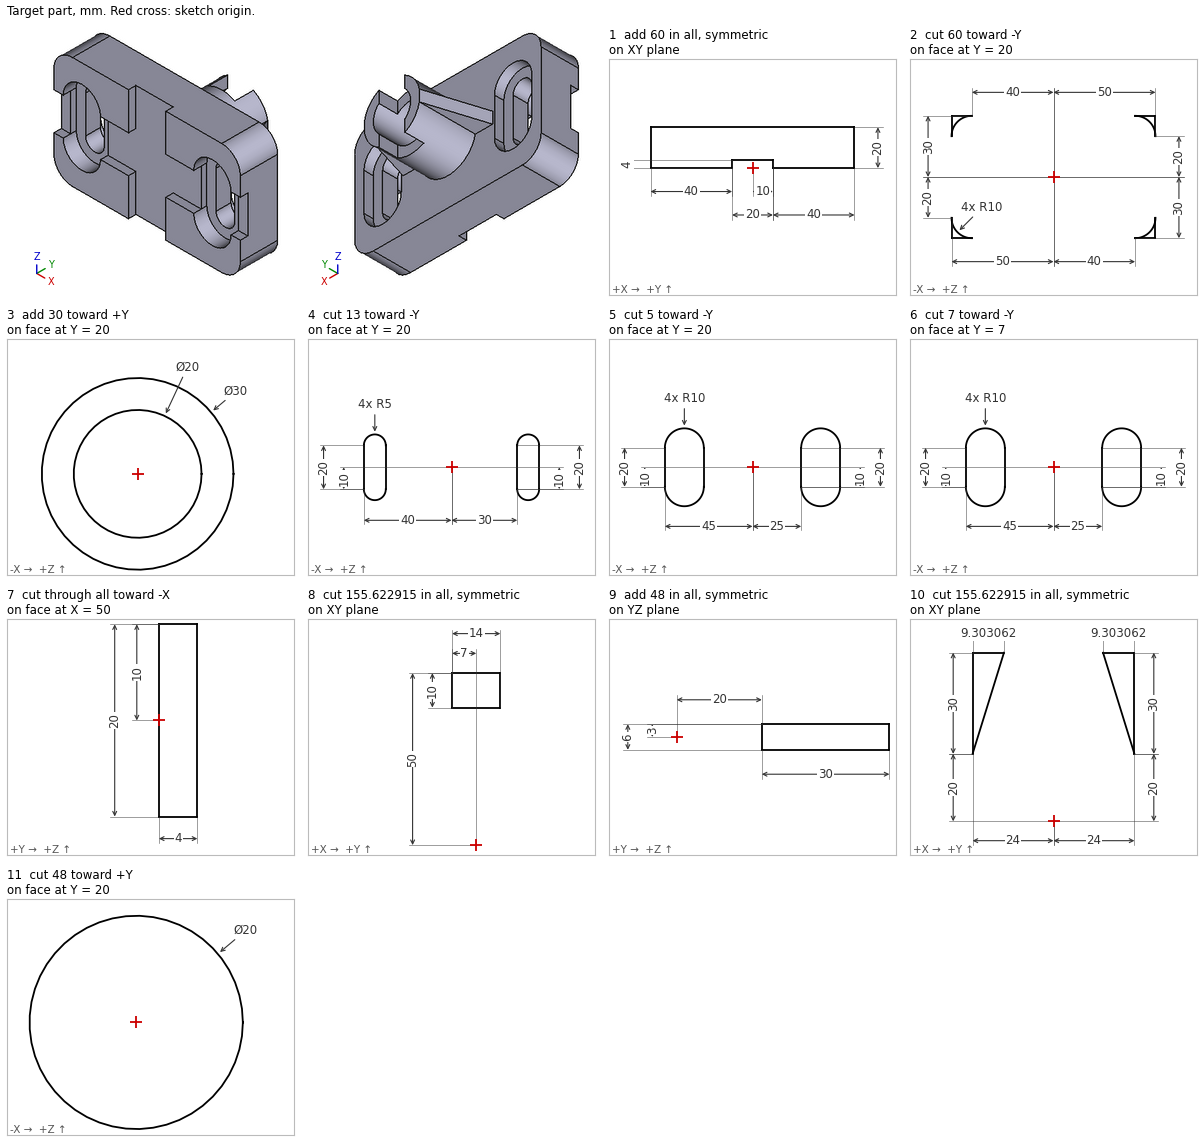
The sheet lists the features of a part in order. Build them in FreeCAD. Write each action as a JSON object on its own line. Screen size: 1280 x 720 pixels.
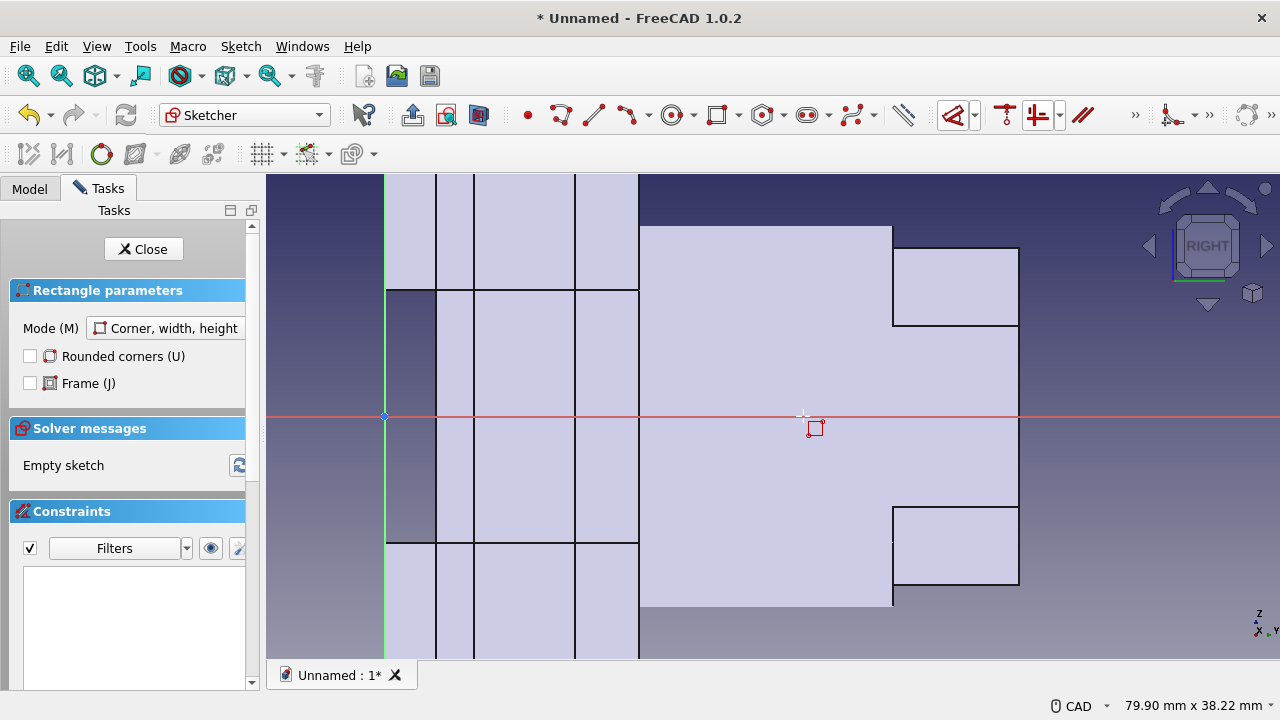
{"action": "left_click", "coordinate": [639, 378]}
{"action": "left_click", "coordinate": [1019, 455]}
{"action": "key", "text": "Escape"}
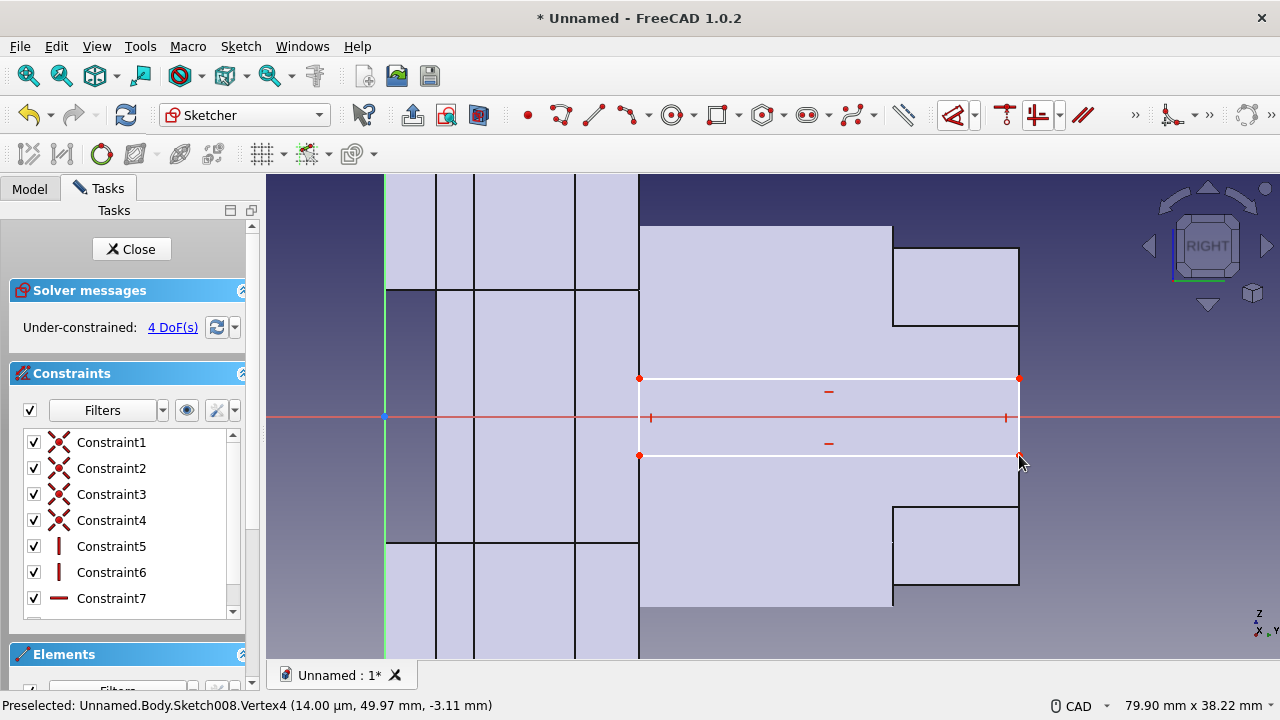
{"action": "left_click", "coordinate": [639, 402]}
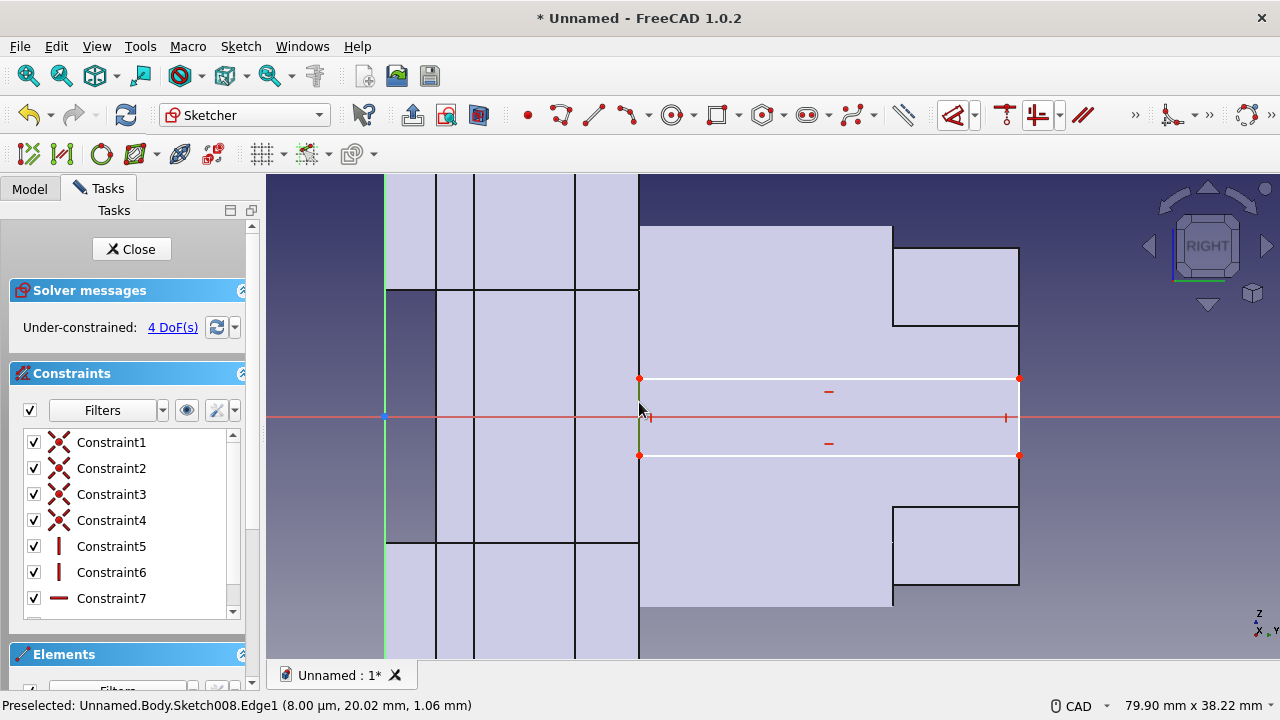
{"action": "key", "text": "i"}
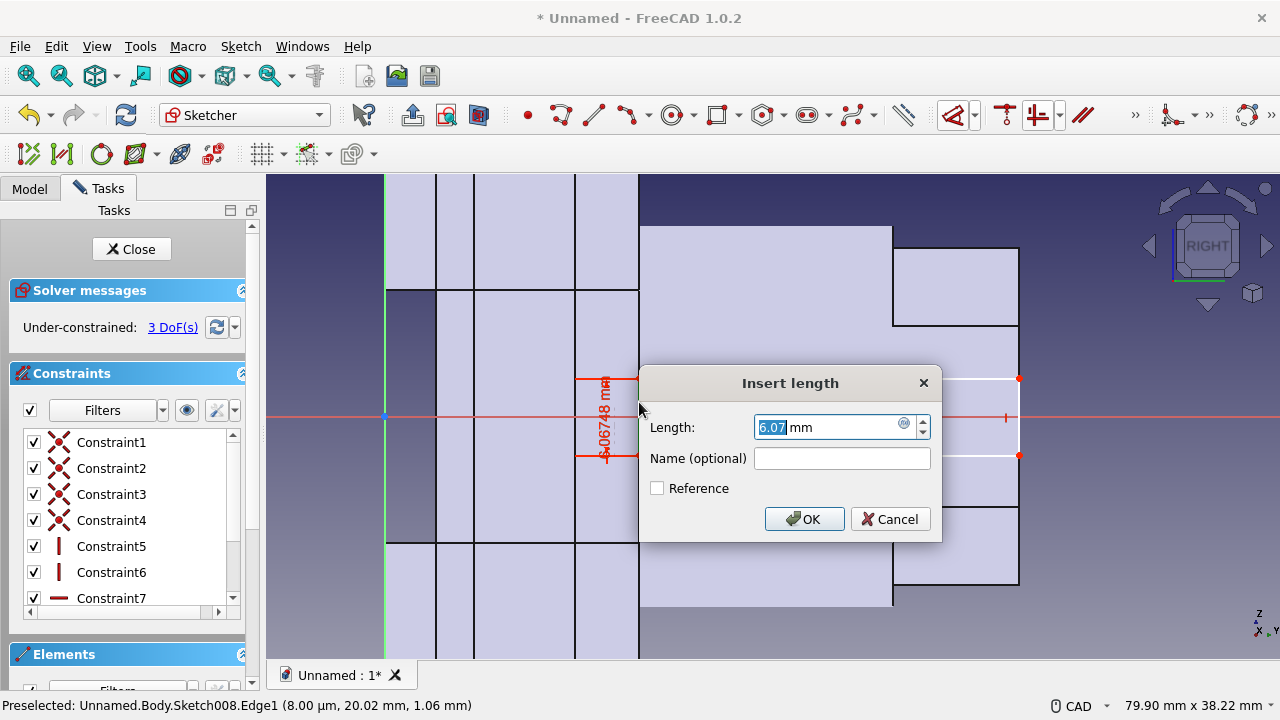
{"action": "type", "text": "6"}
{"action": "key", "text": "Return"}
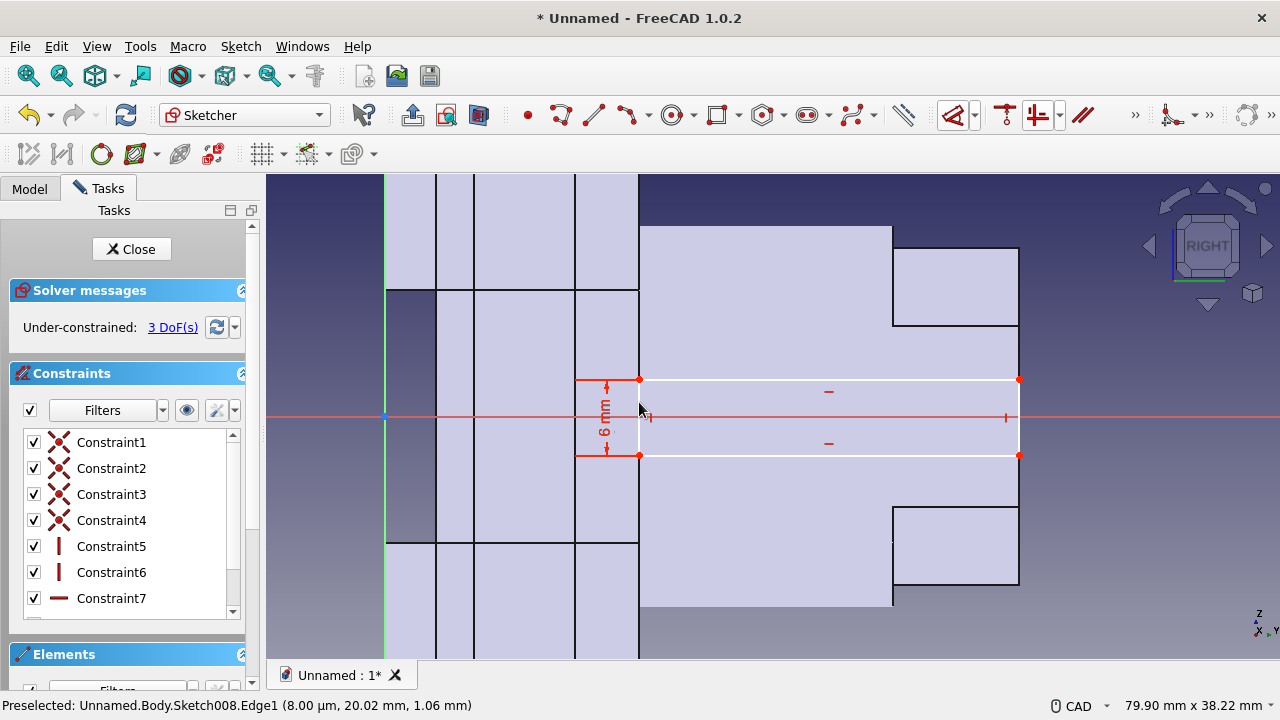
{"action": "left_click", "coordinate": [753, 456]}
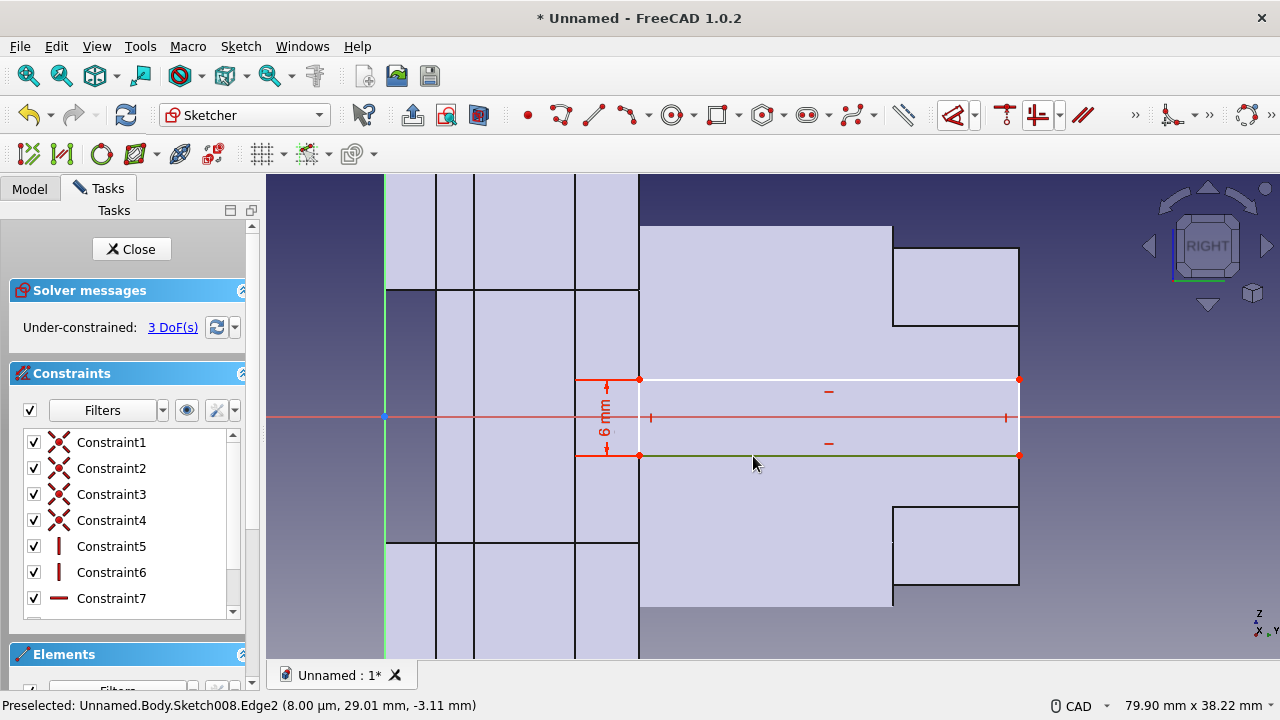
{"action": "key", "text": "l"}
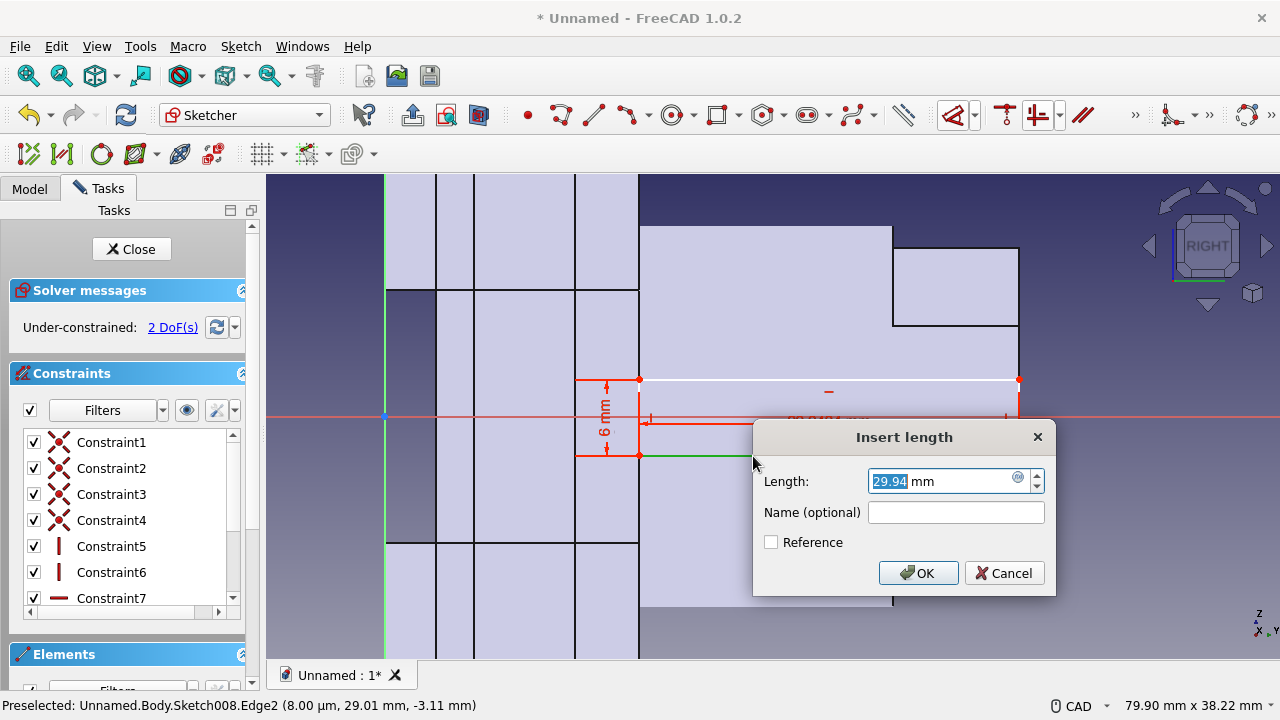
{"action": "type", "text": "30"}
{"action": "key", "text": "Return"}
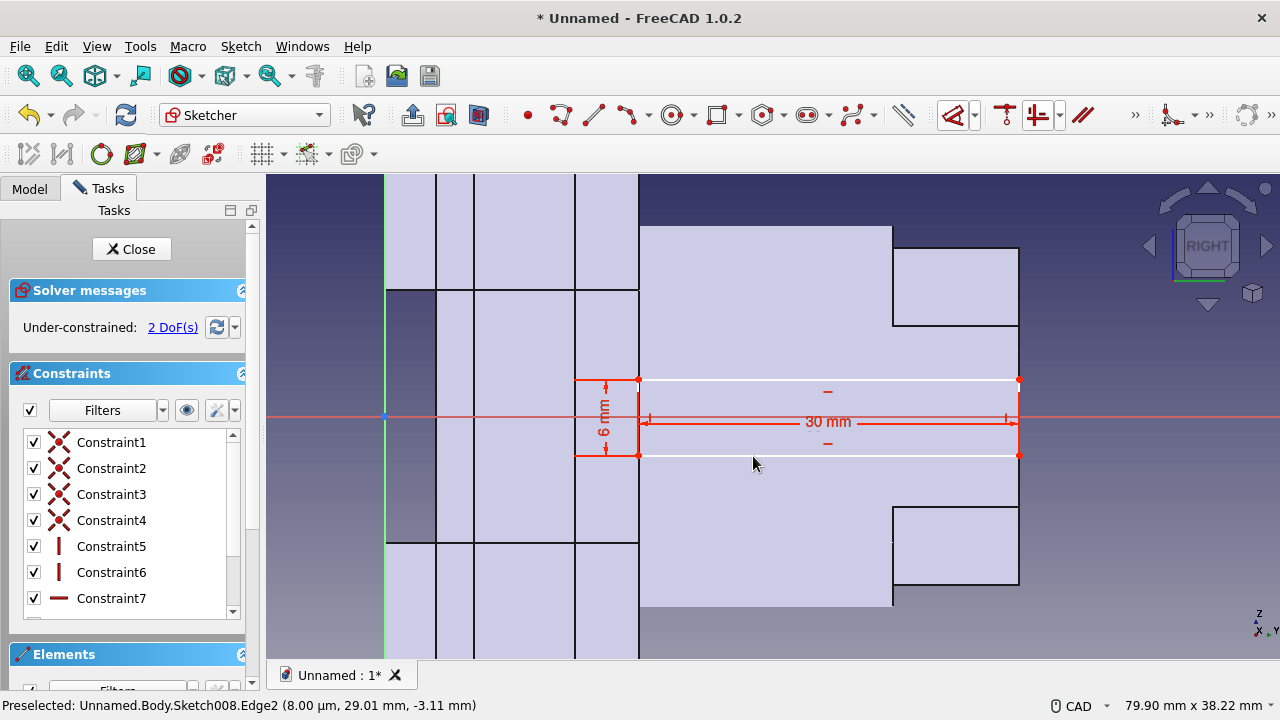
{"action": "left_click", "coordinate": [638, 380]}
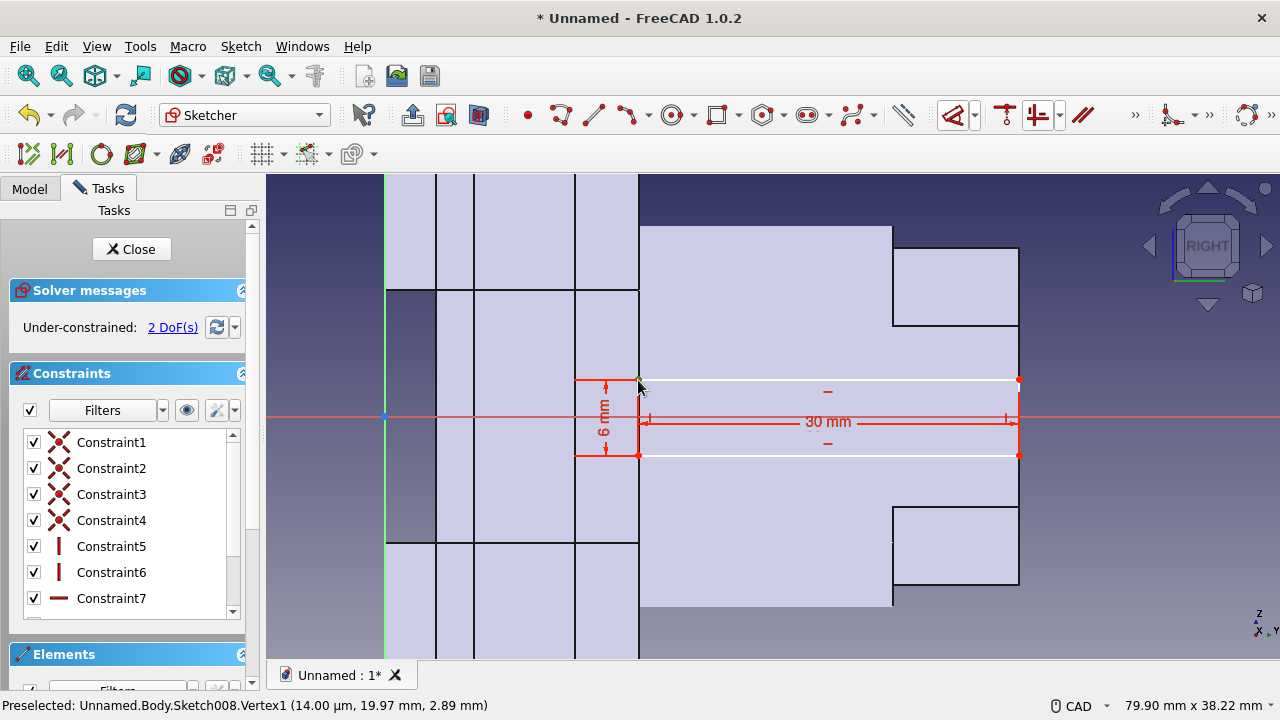
{"action": "key", "text": "i"}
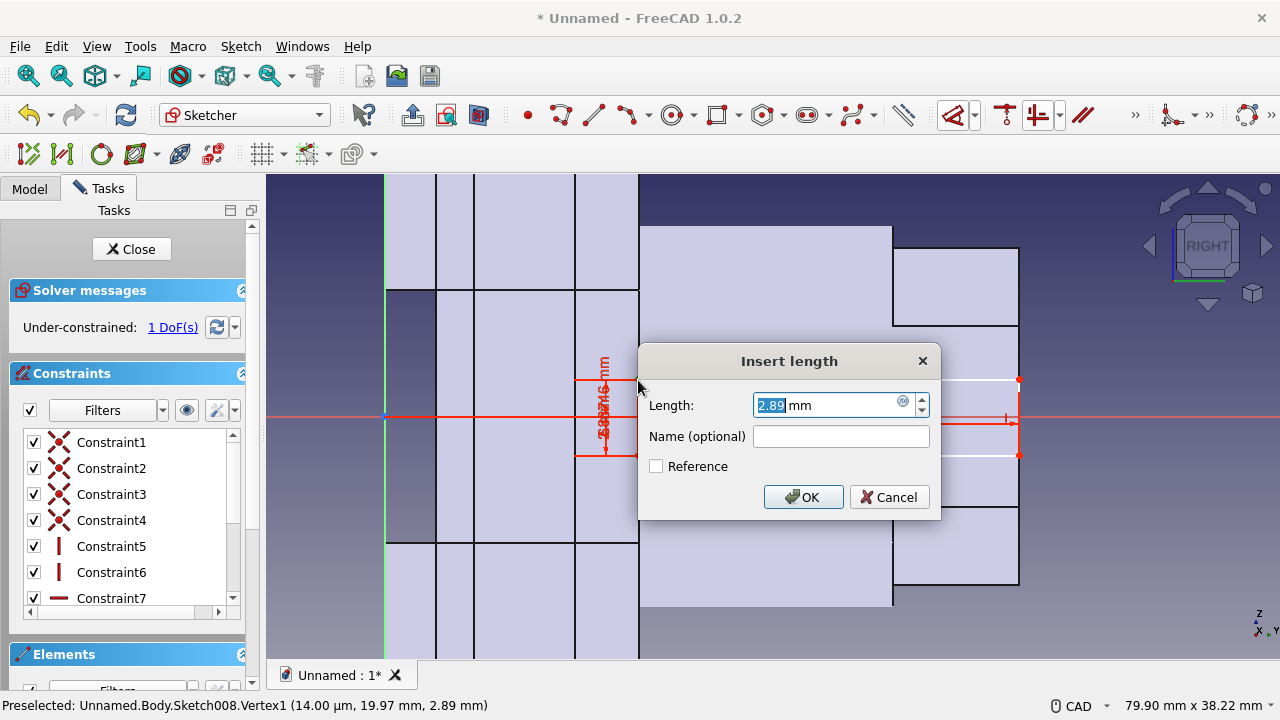
{"action": "type", "text": "3"}
{"action": "key", "text": "Return"}